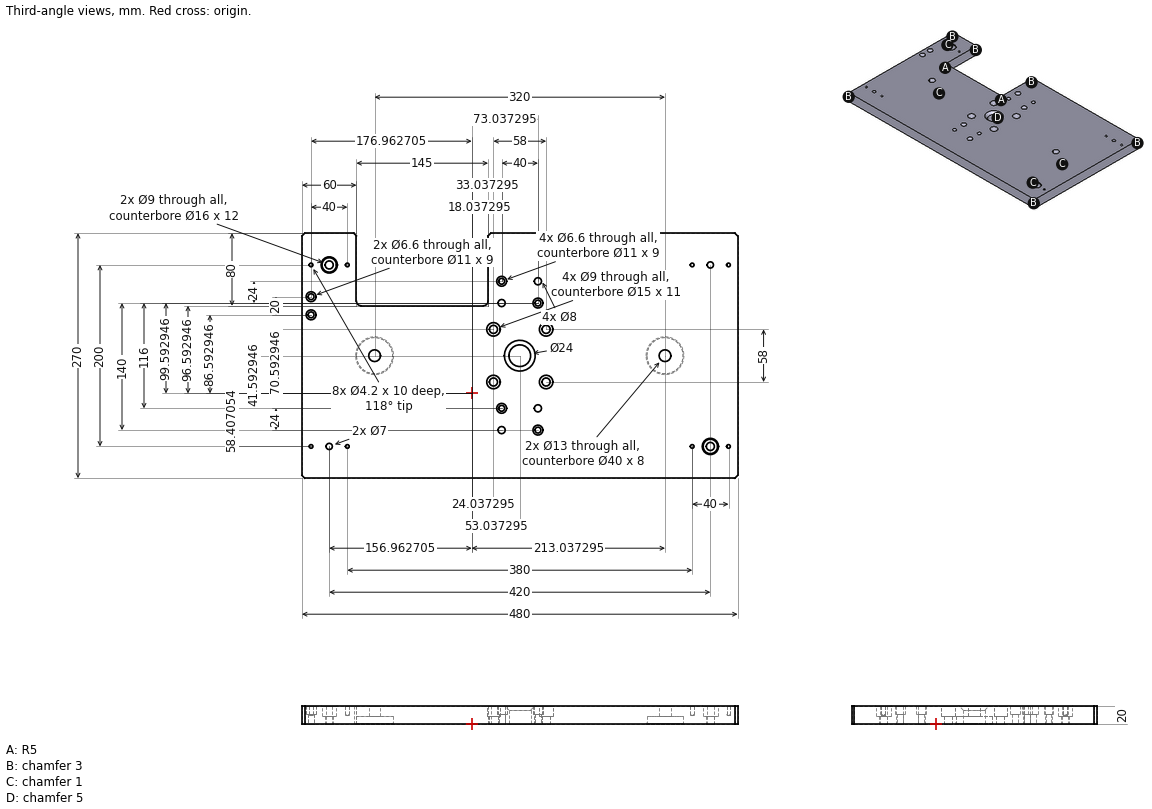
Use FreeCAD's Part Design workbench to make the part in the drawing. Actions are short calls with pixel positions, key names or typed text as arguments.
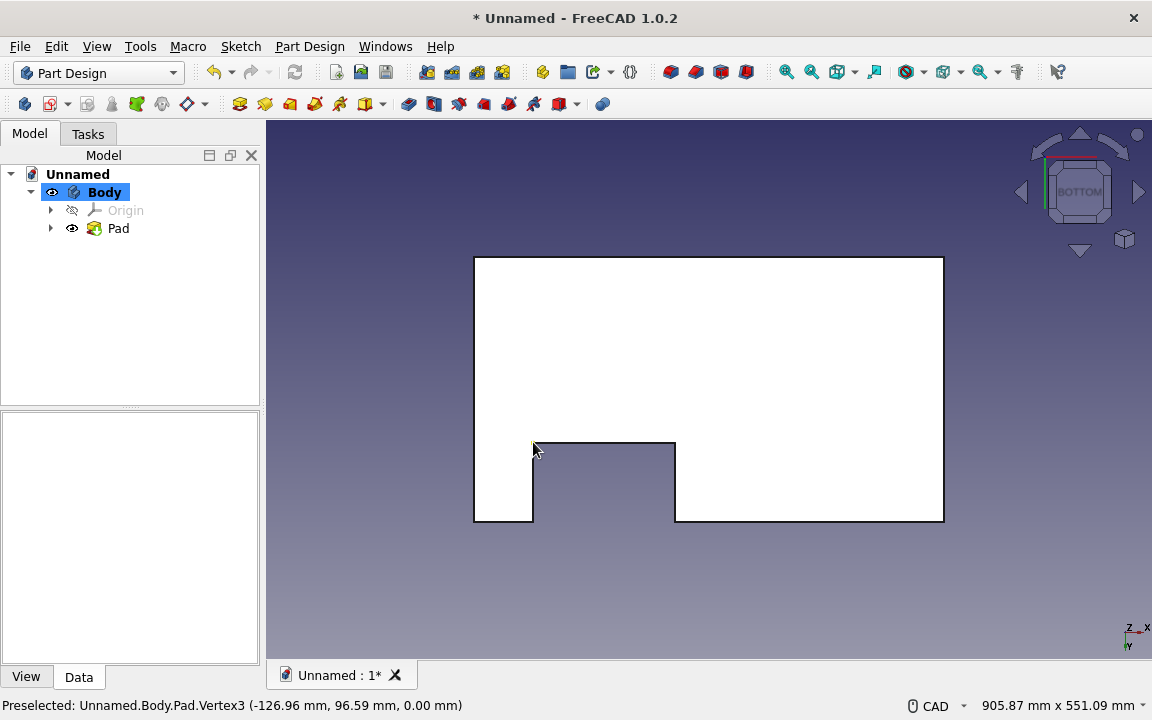
key(4)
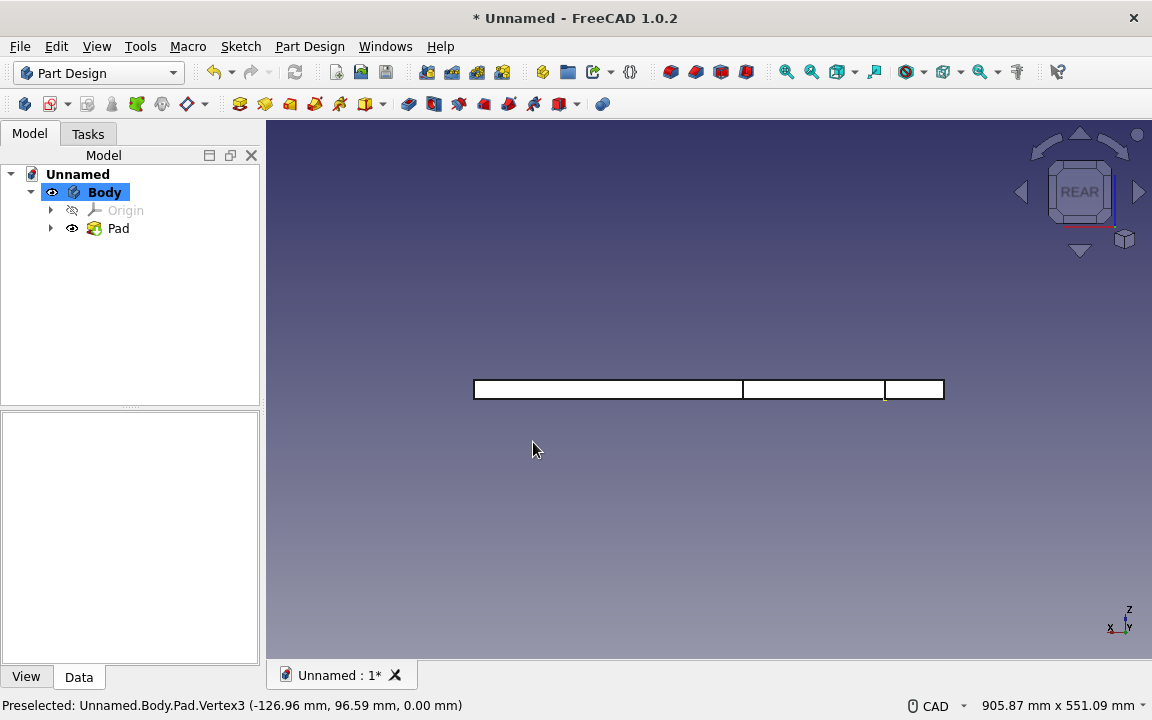
scroll(885, 388, up, 4)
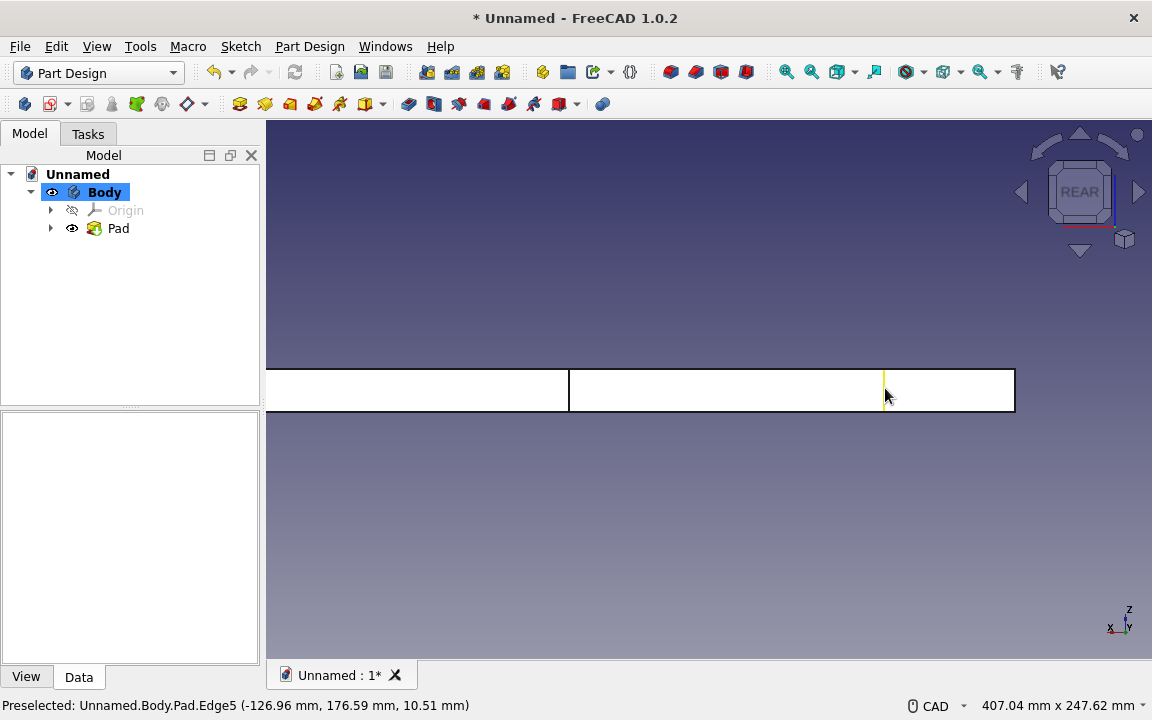
key(v)
key(f)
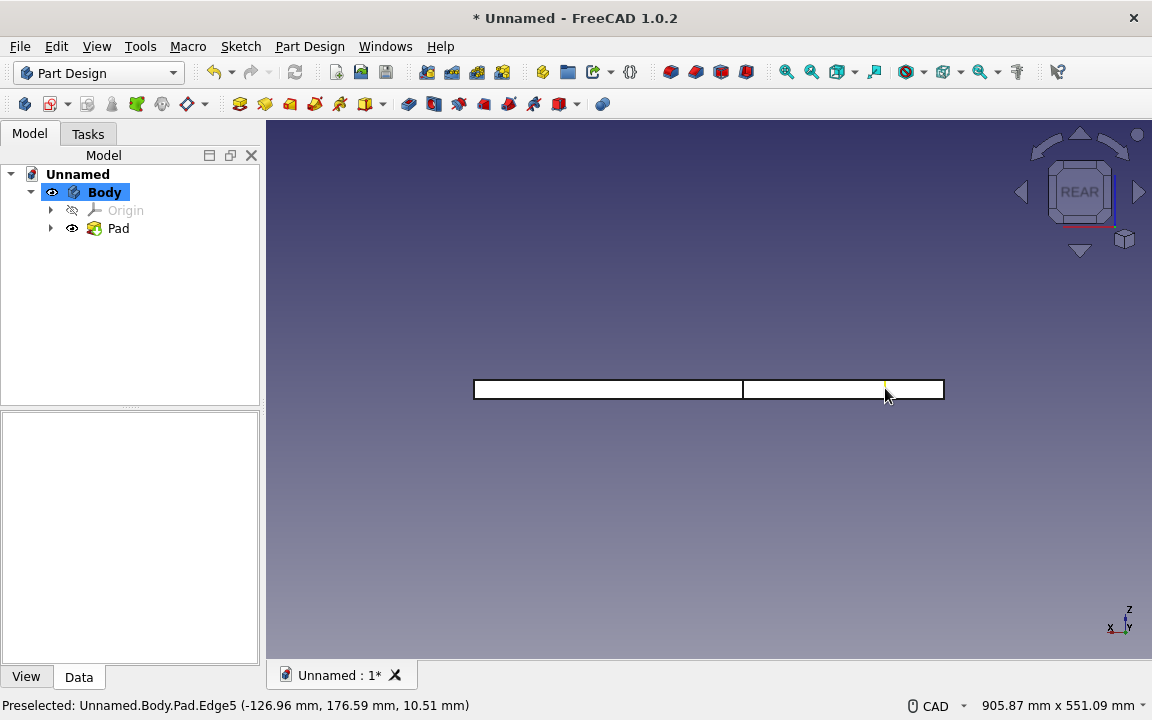
key(6)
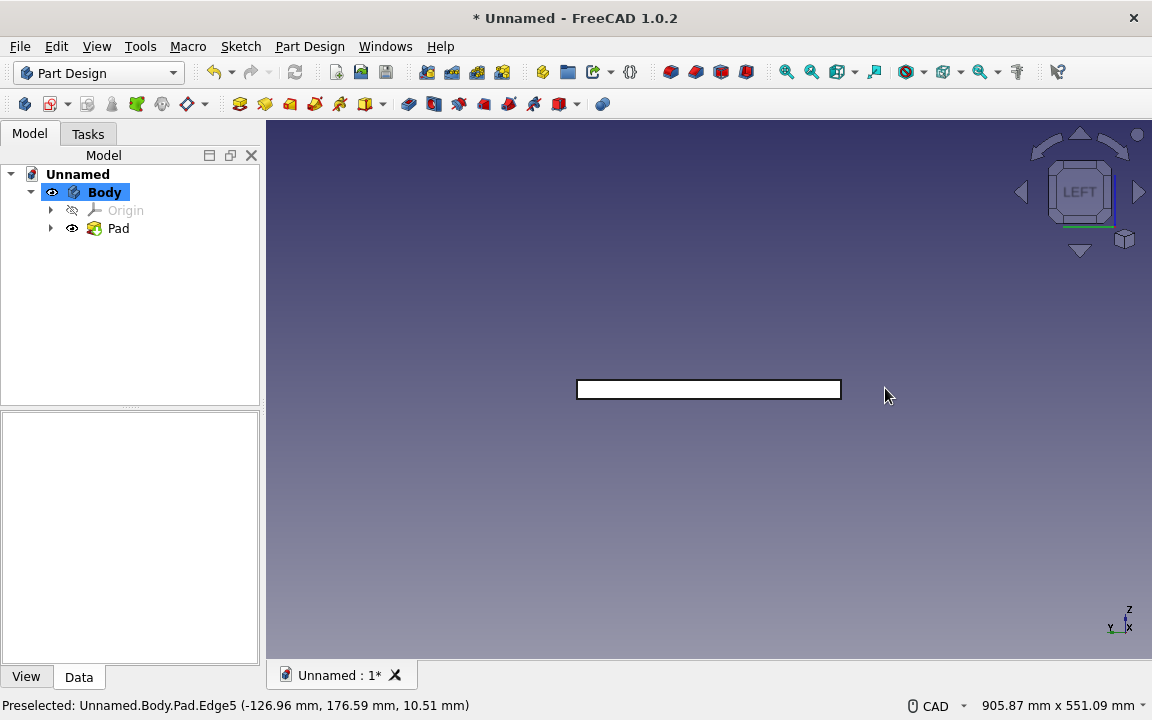
key(v)
key(f)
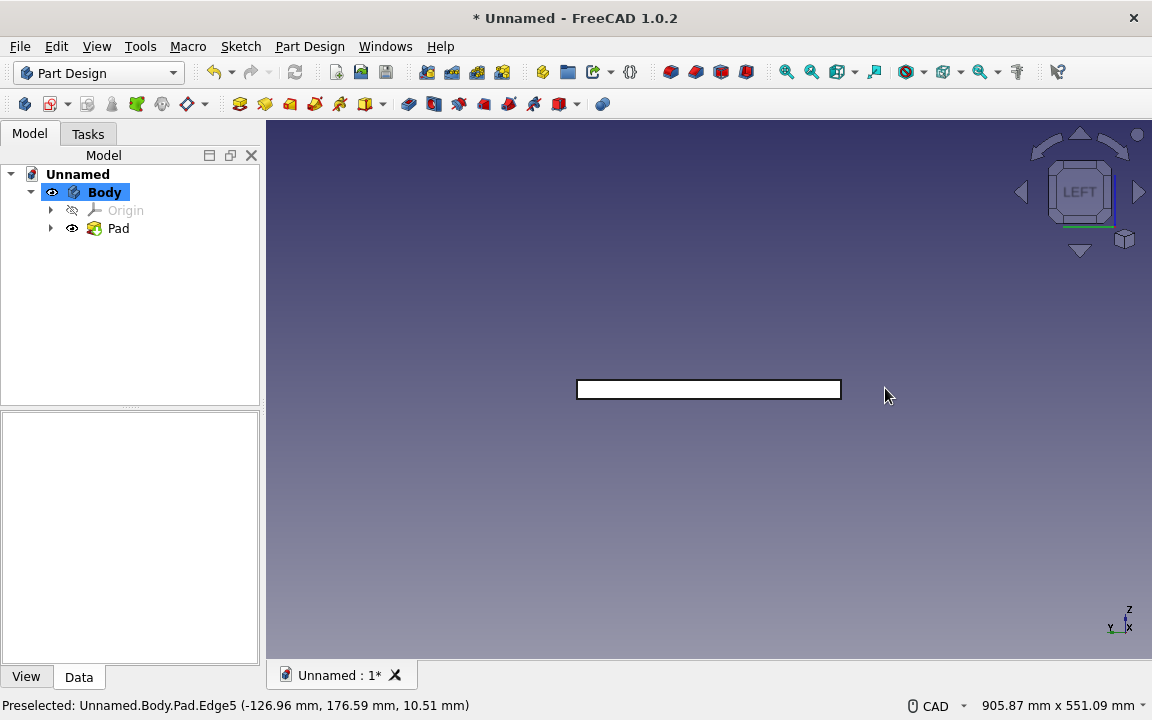
scroll(655, 388, up, 4)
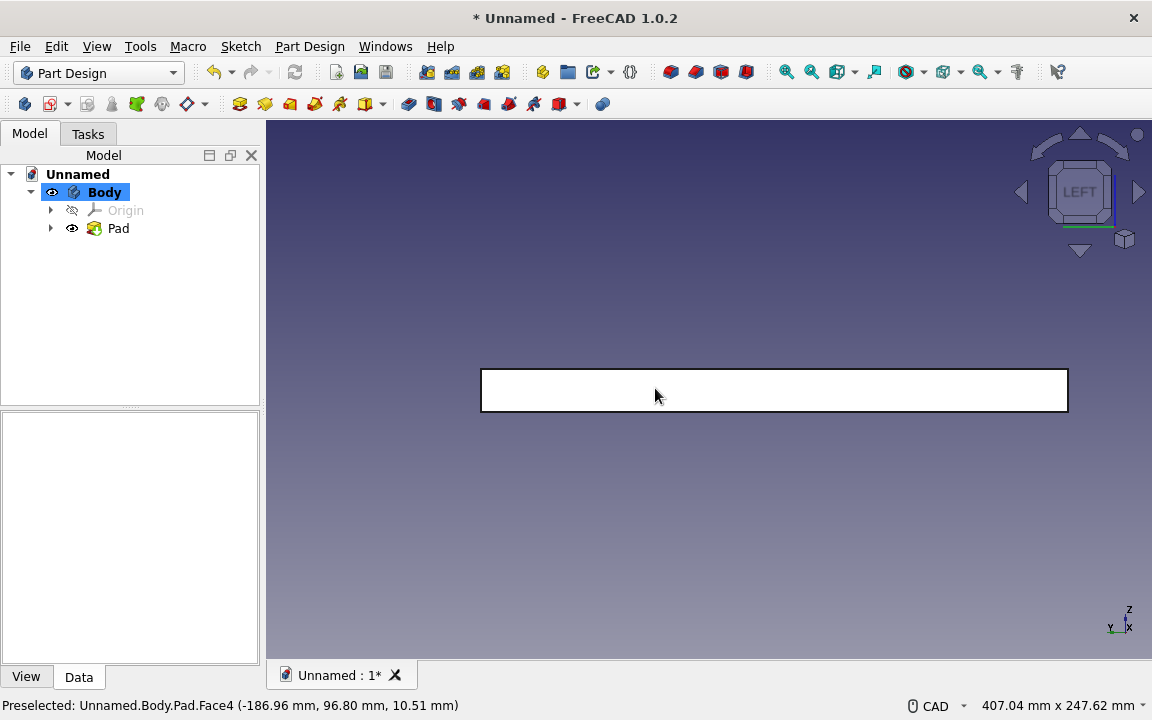
click(787, 72)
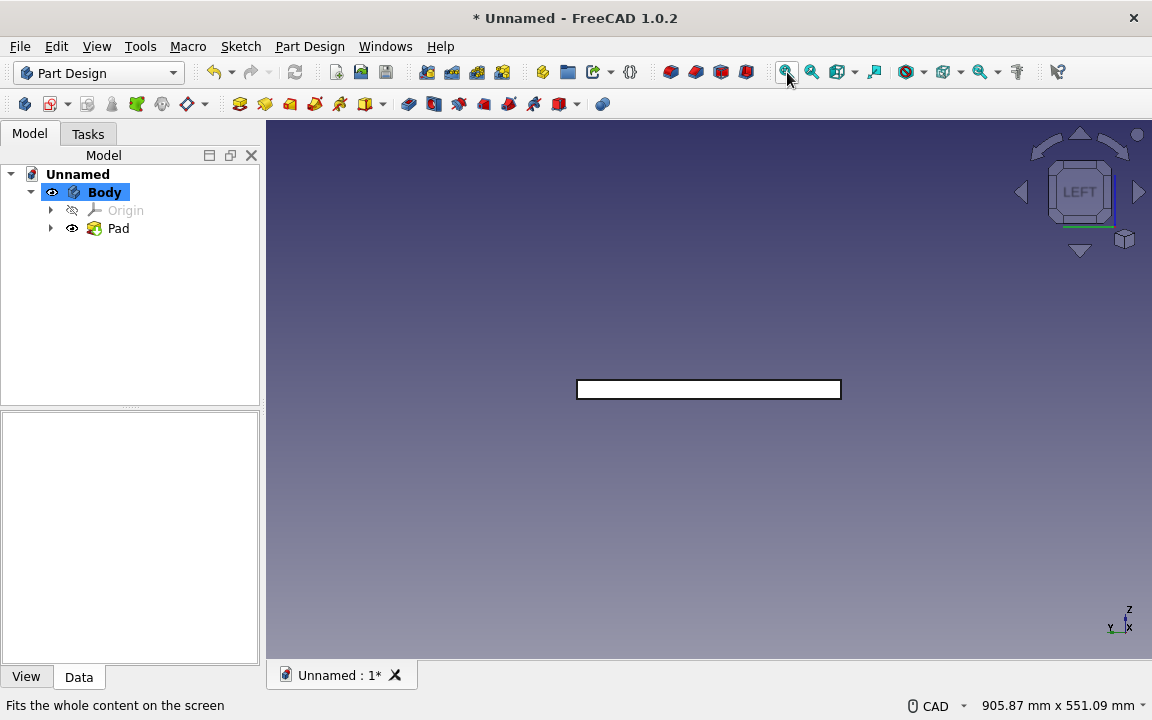
key(v)
key(3)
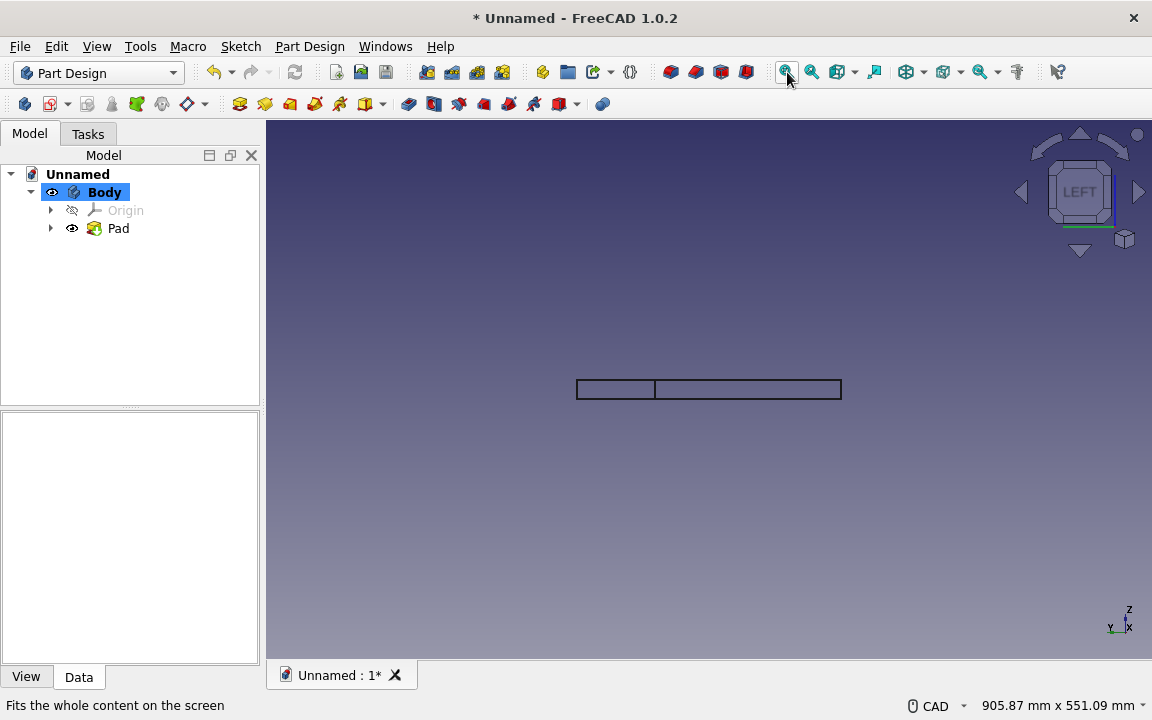
key(0)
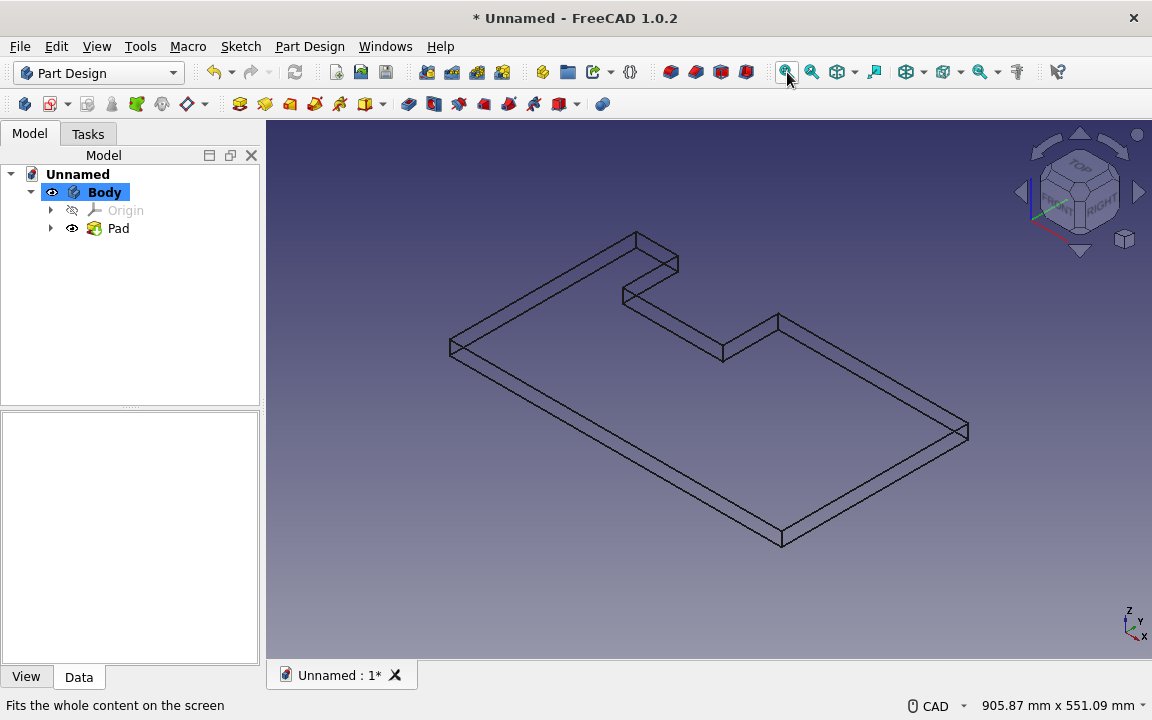
click(623, 295)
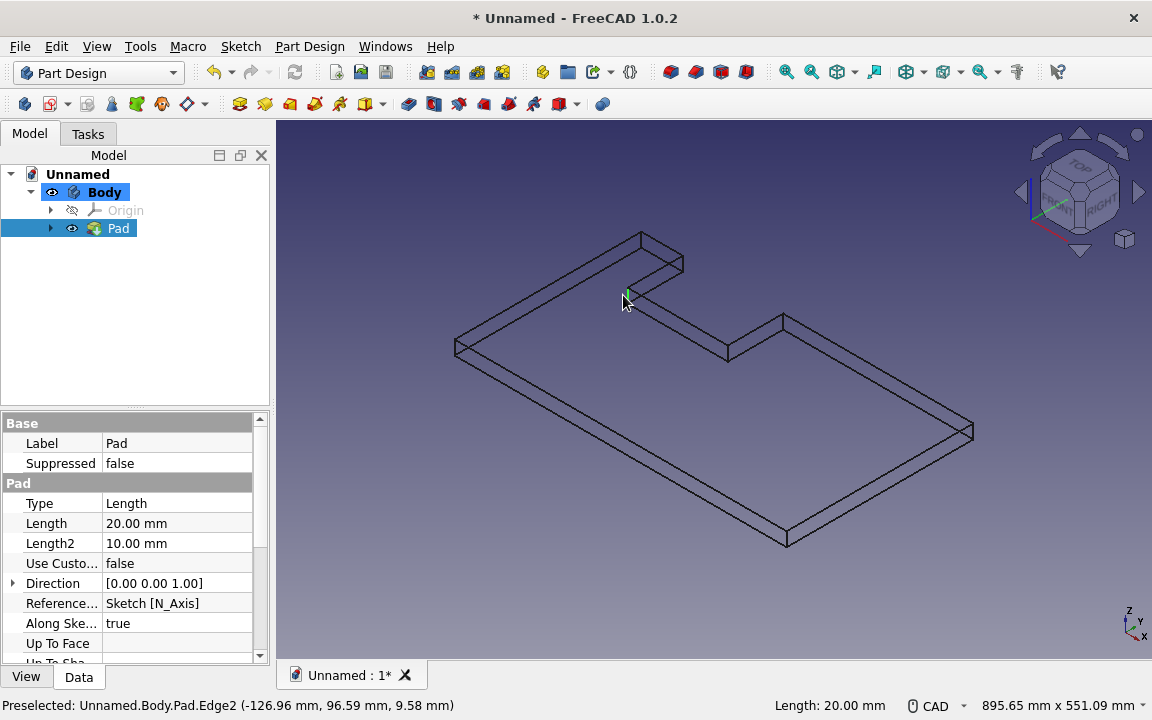
click(728, 353, ctrl)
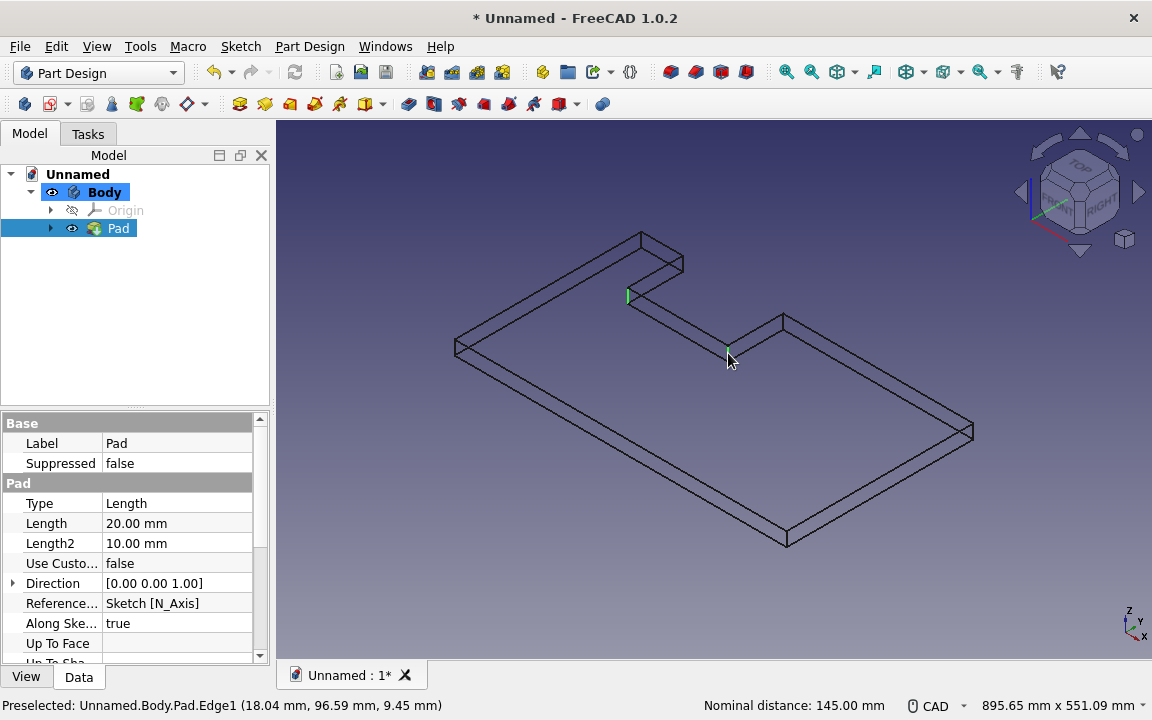
key(v)
key(1)